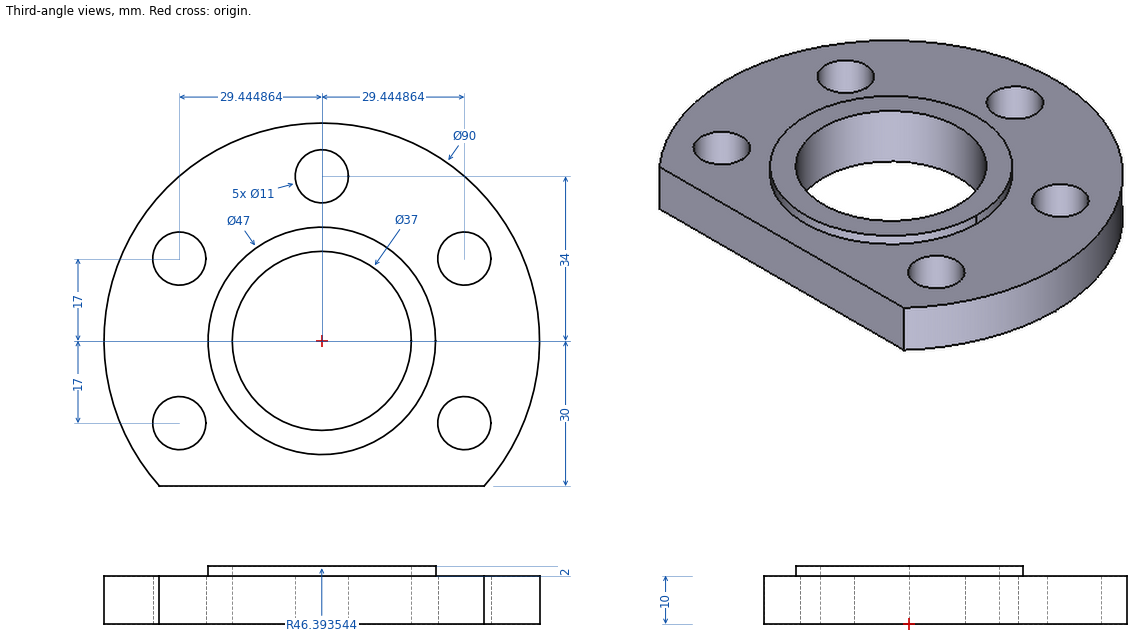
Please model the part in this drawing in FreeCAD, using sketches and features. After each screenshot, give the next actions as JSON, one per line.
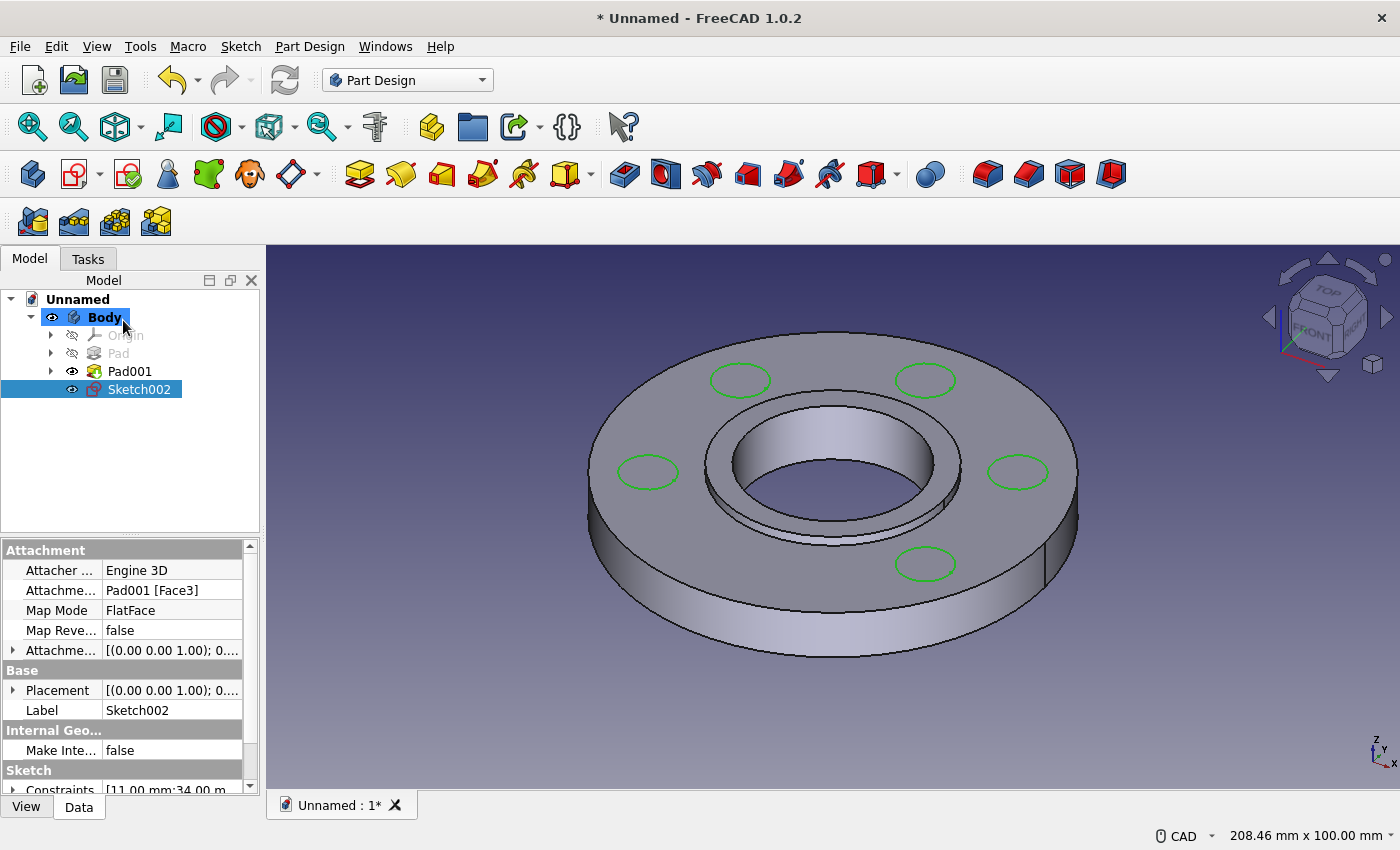
{"action": "left_click", "coordinate": [625, 174]}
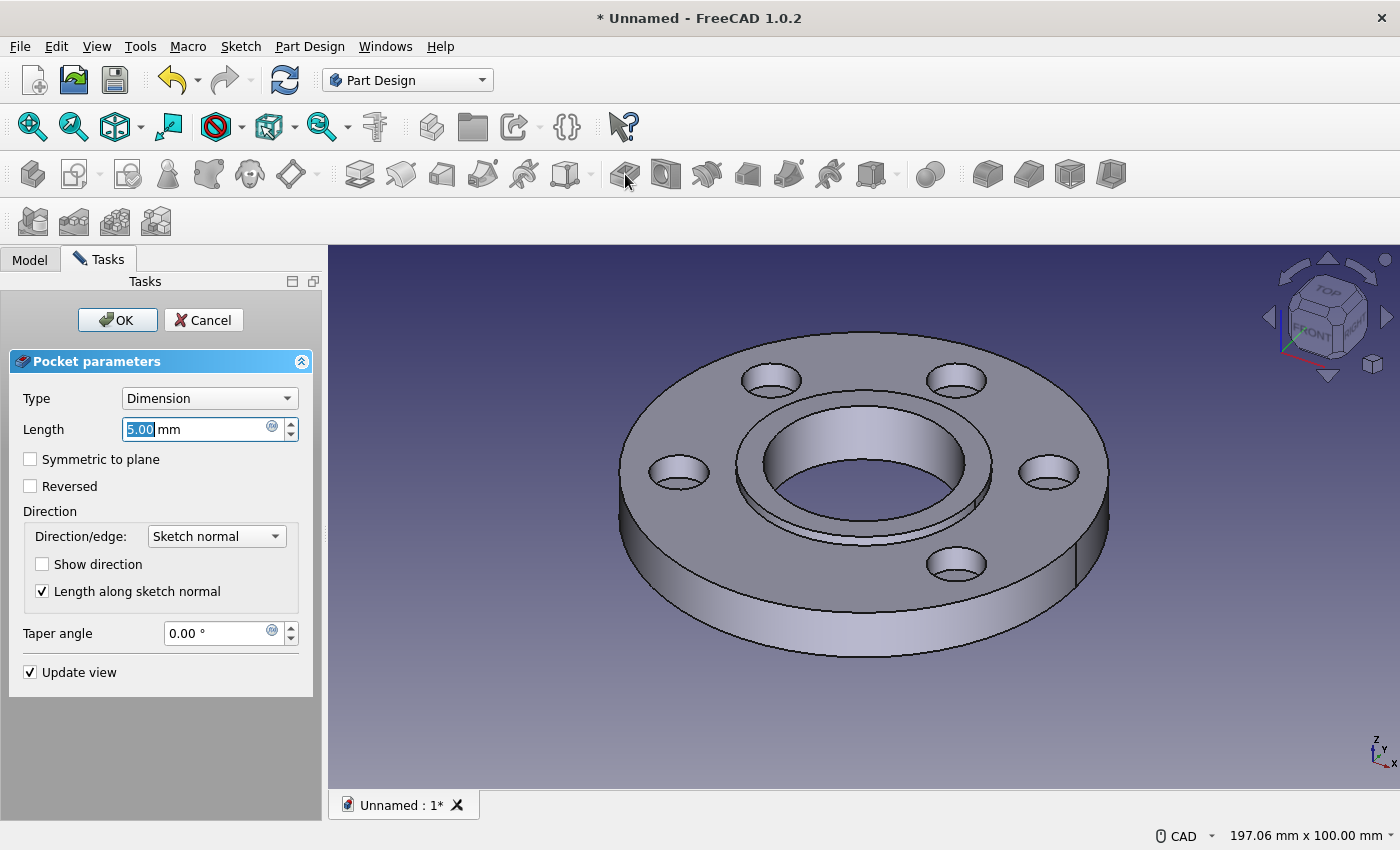
{"action": "left_click", "coordinate": [210, 398]}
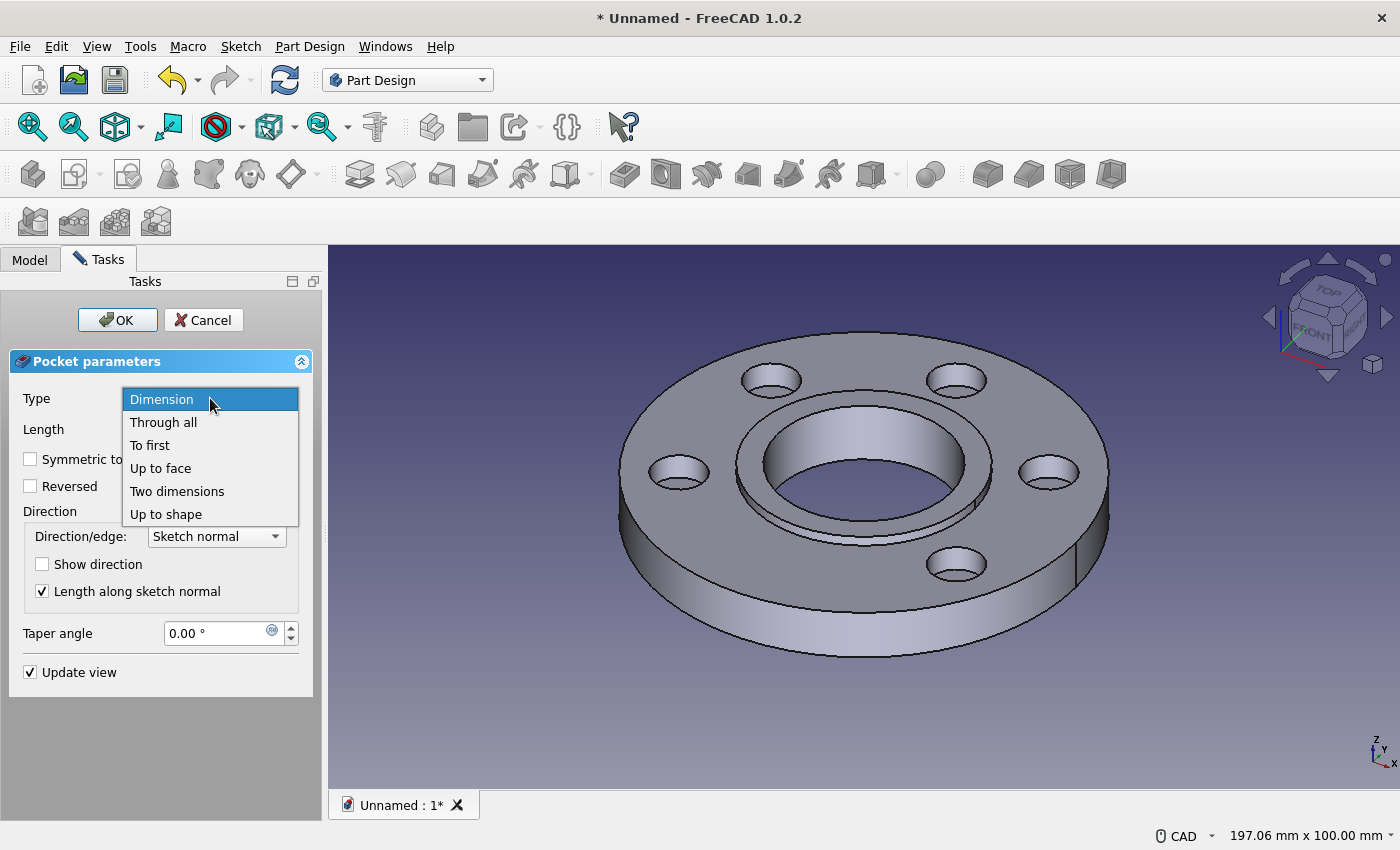
{"action": "left_click", "coordinate": [208, 422]}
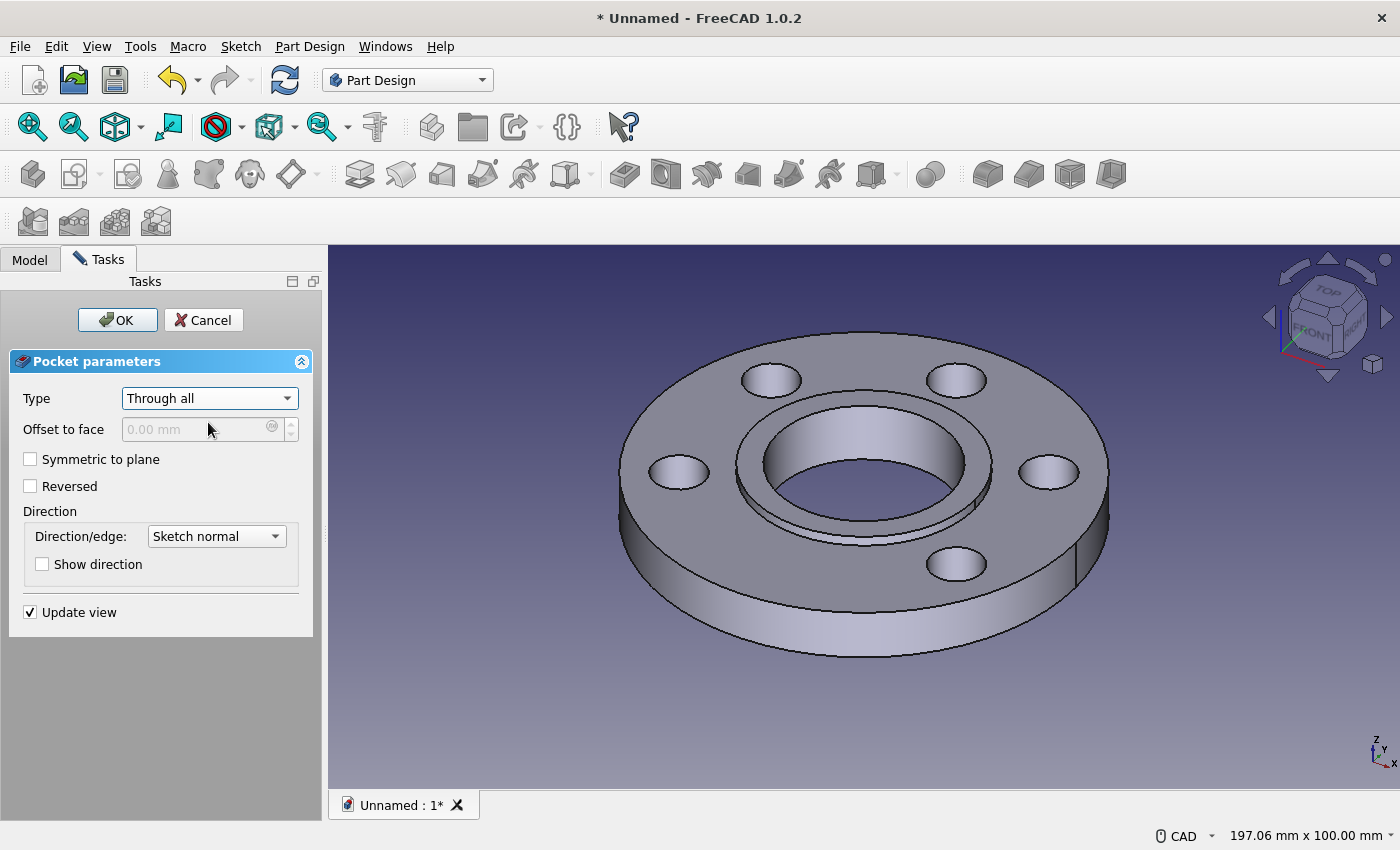
{"action": "left_click", "coordinate": [118, 320]}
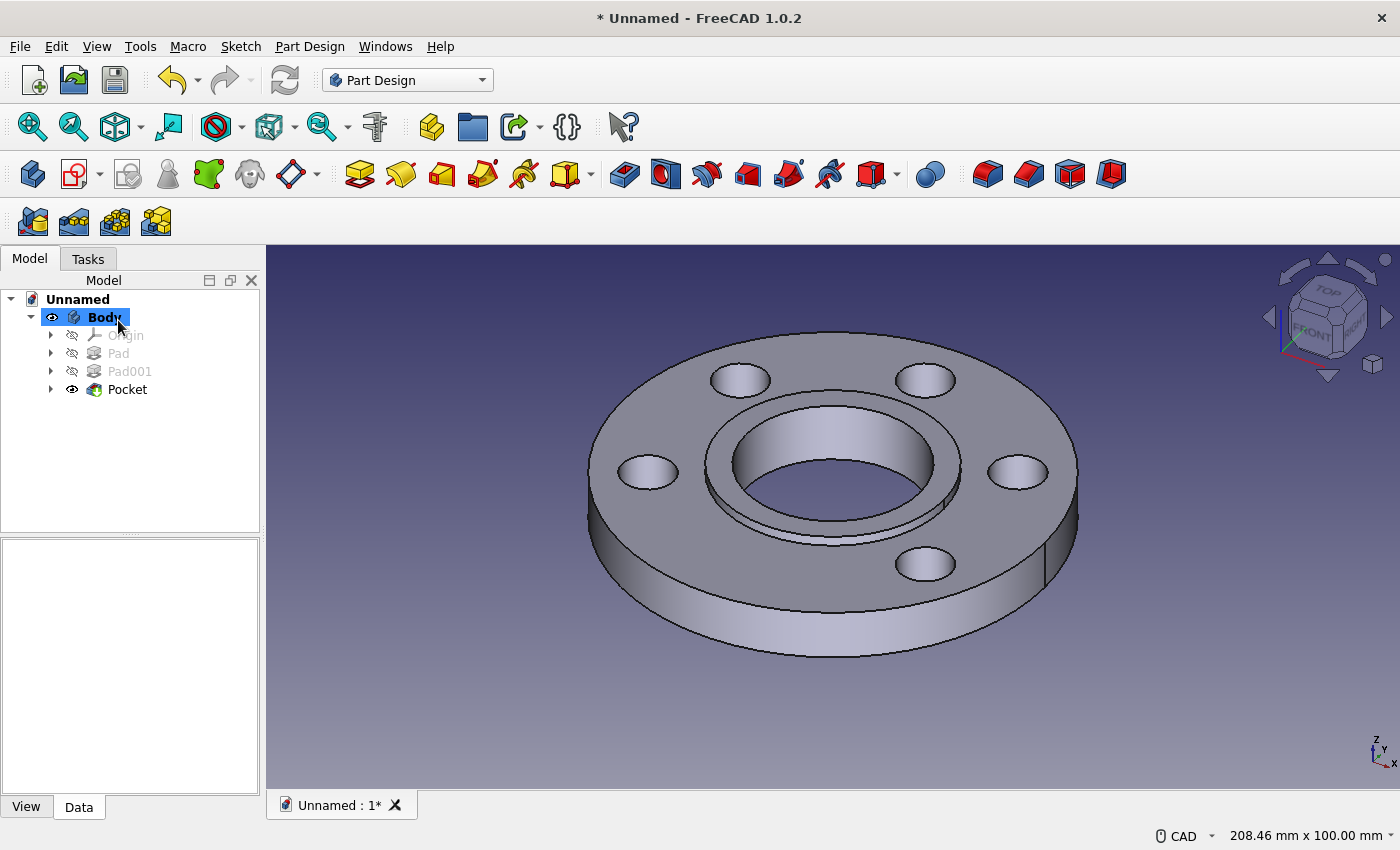
{"action": "left_click", "coordinate": [1015, 532]}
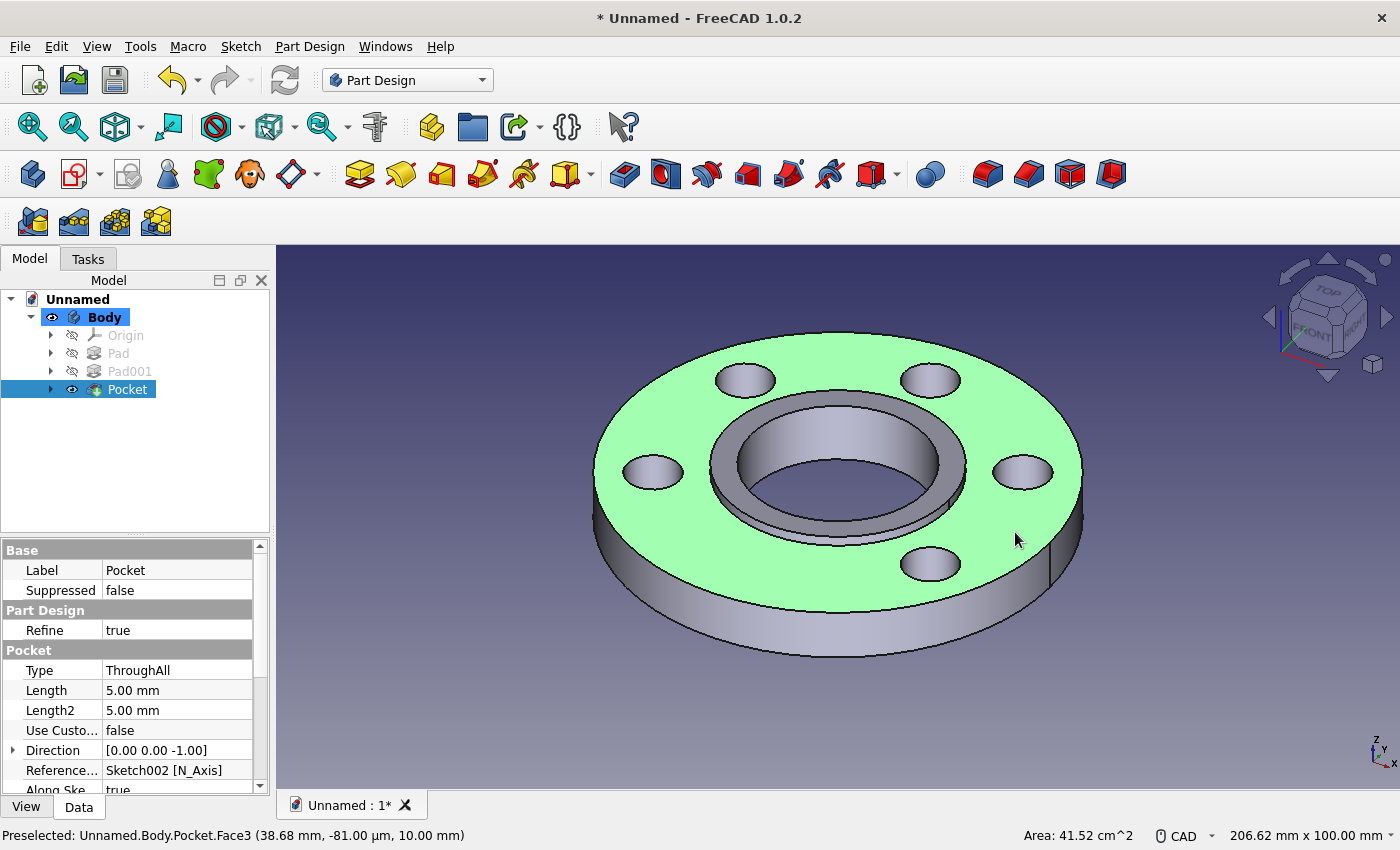
{"action": "left_click", "coordinate": [74, 174]}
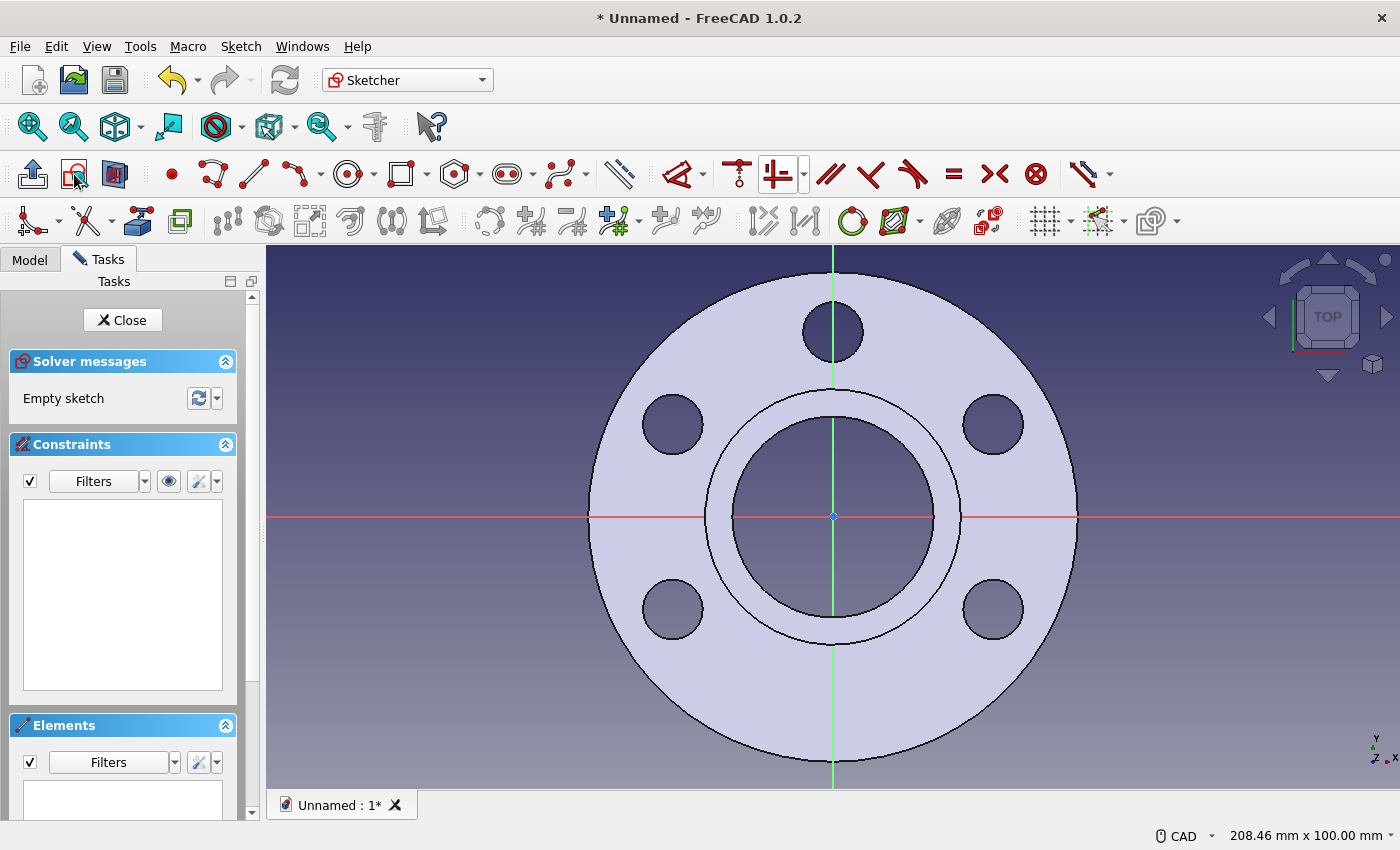
{"action": "scroll", "coordinate": [455, 273], "scroll_direction": "down", "scroll_amount": 1}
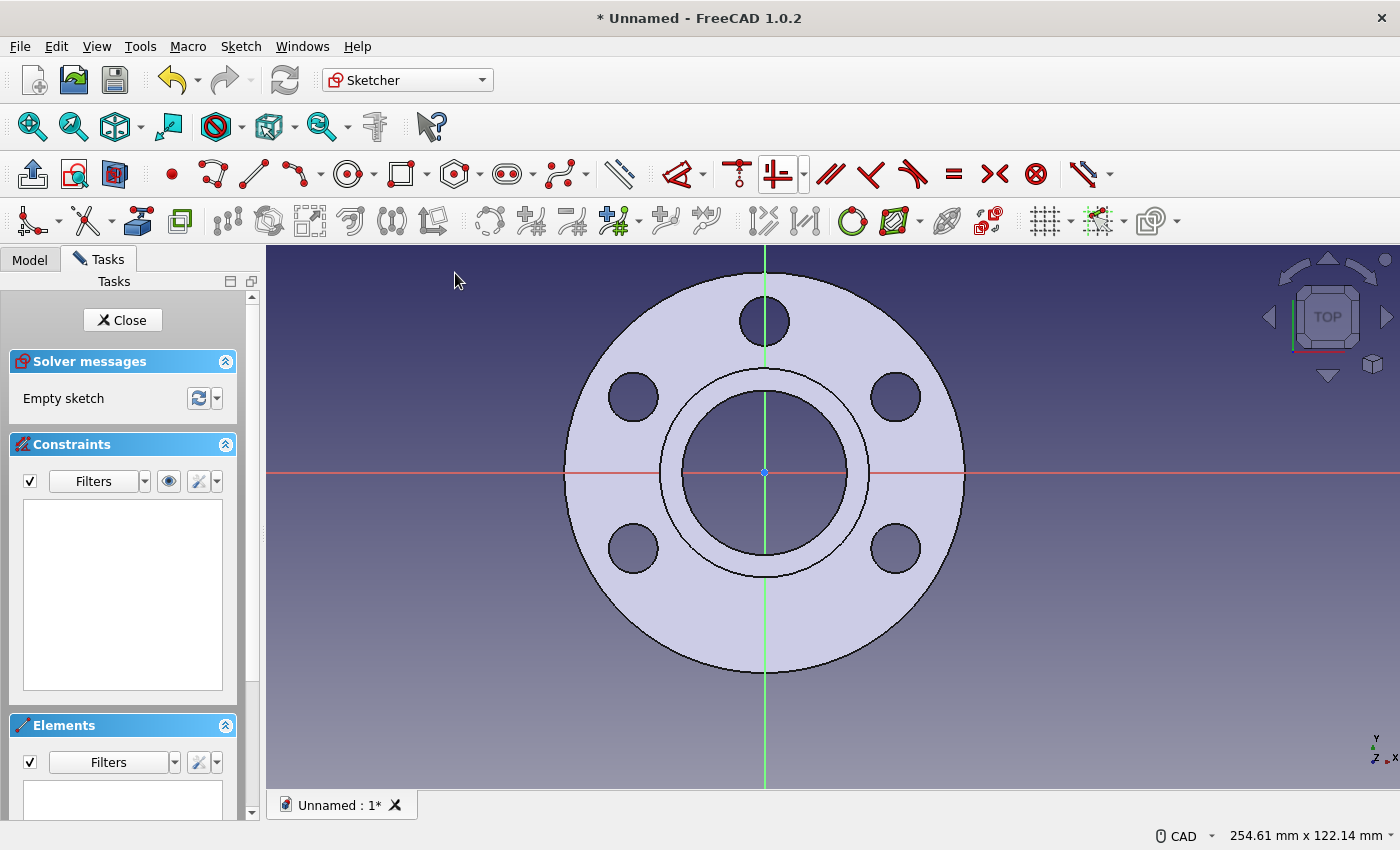
{"action": "scroll", "coordinate": [765, 648], "scroll_direction": "up", "scroll_amount": 3}